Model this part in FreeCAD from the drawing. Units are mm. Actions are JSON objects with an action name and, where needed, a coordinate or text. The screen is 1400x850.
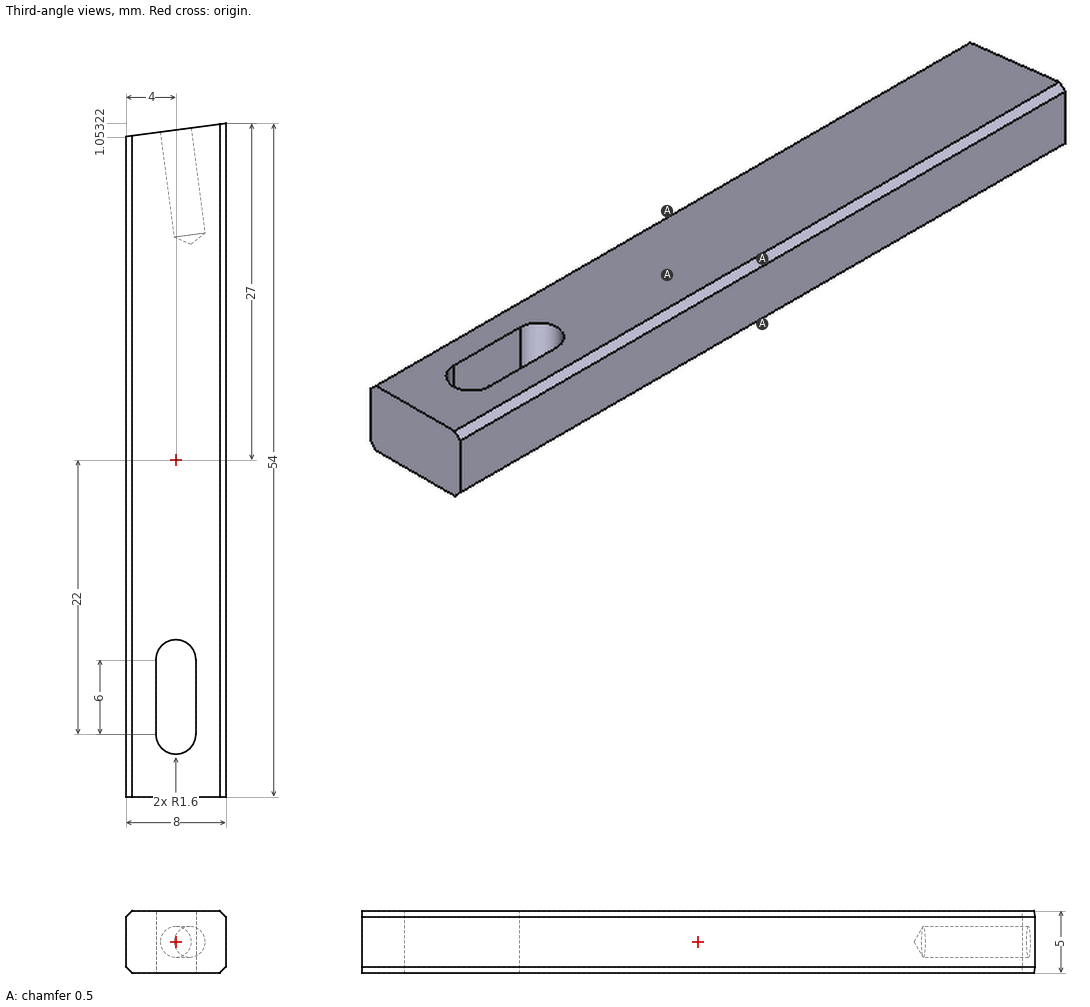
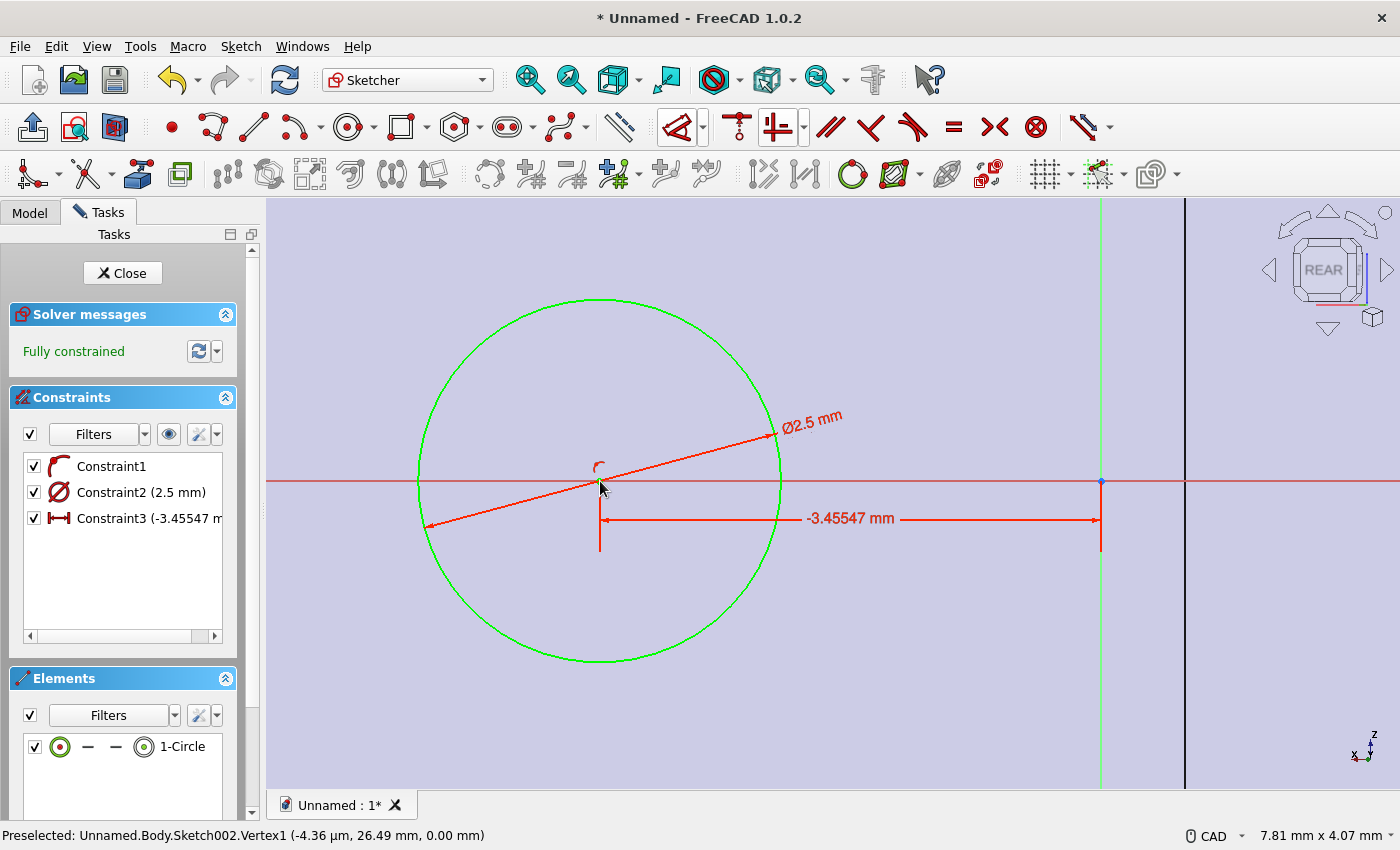
{"action": "left_click", "coordinate": [123, 273]}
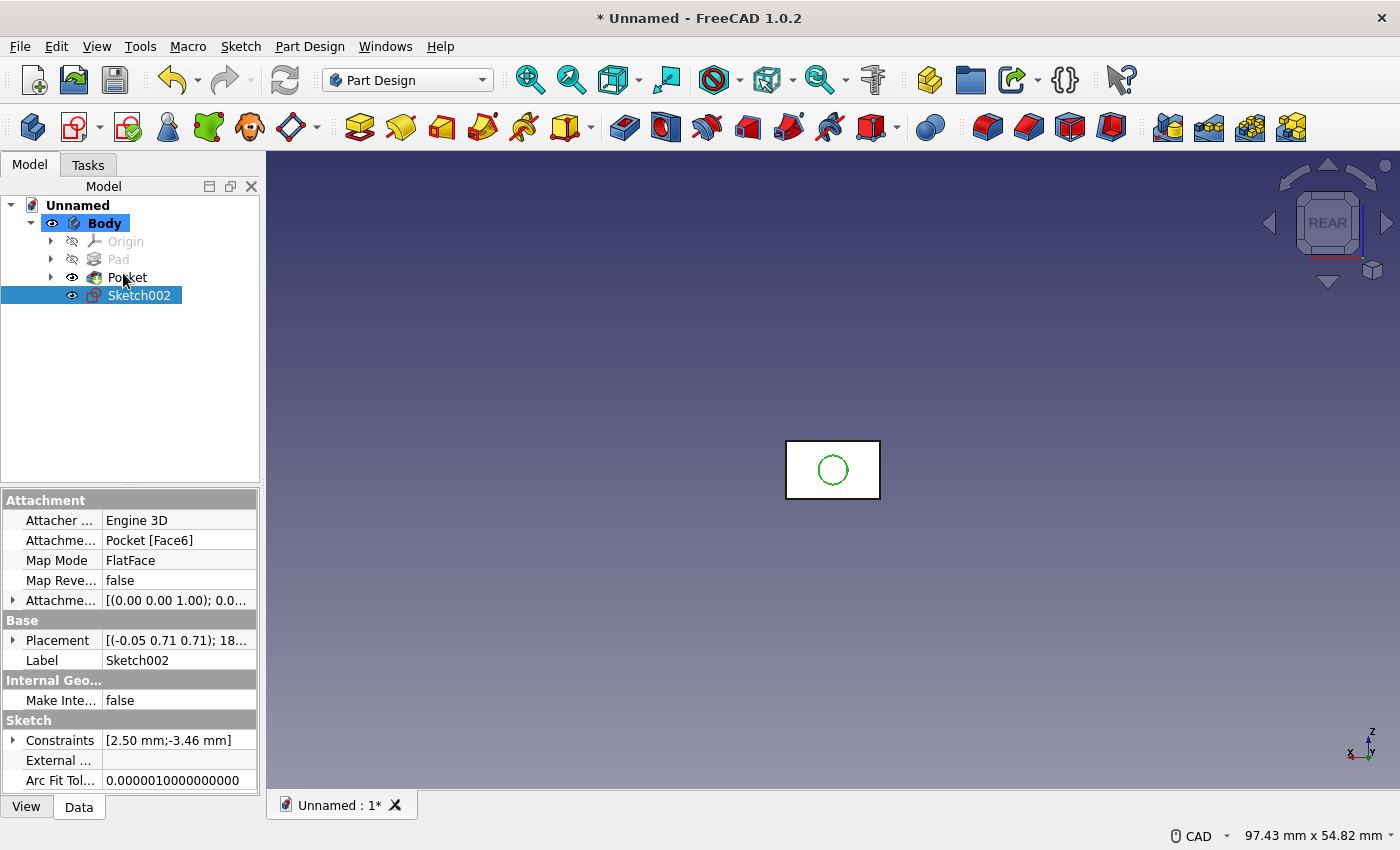
{"action": "left_click", "coordinate": [666, 128]}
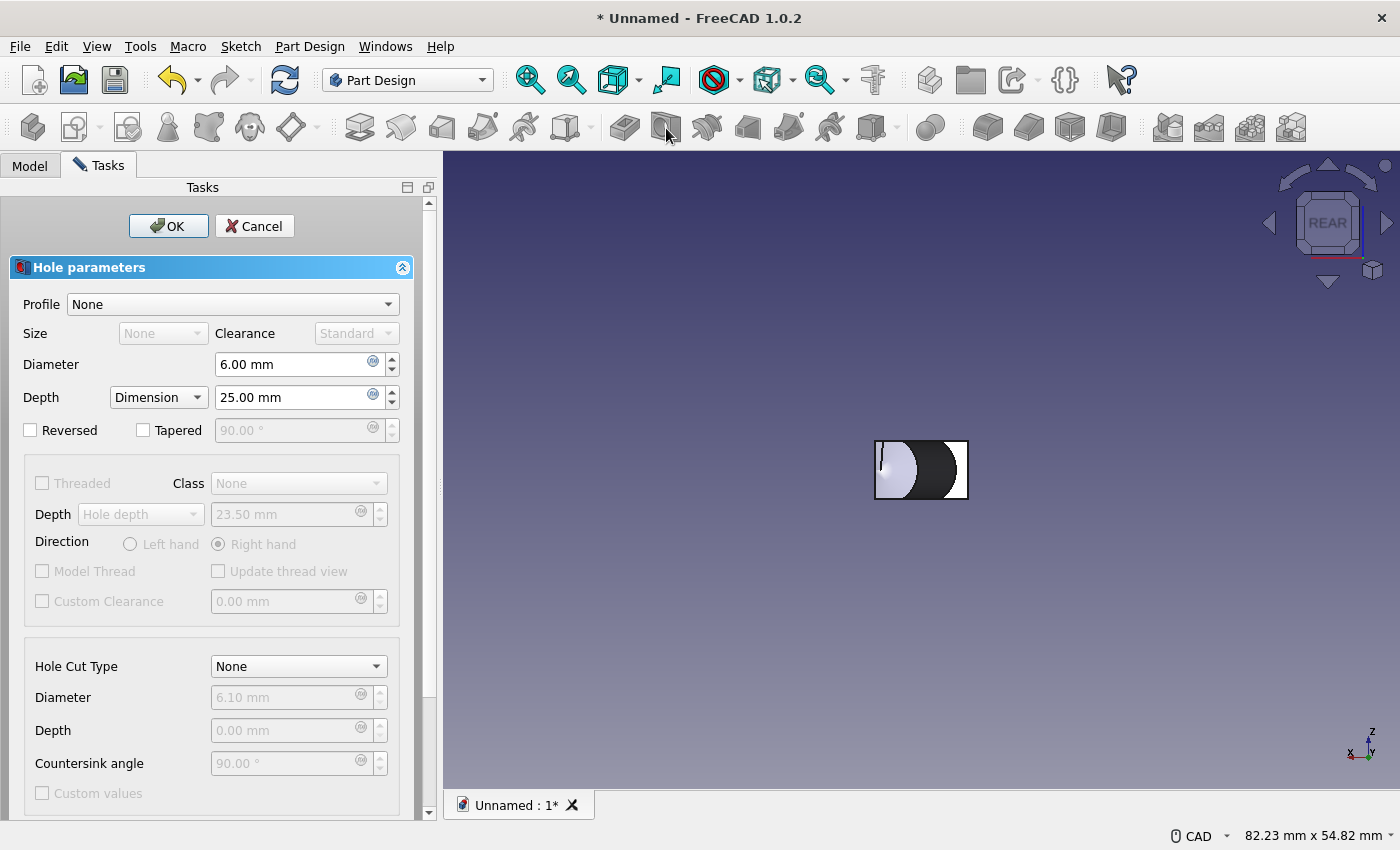
{"action": "triple_click", "coordinate": [300, 364]}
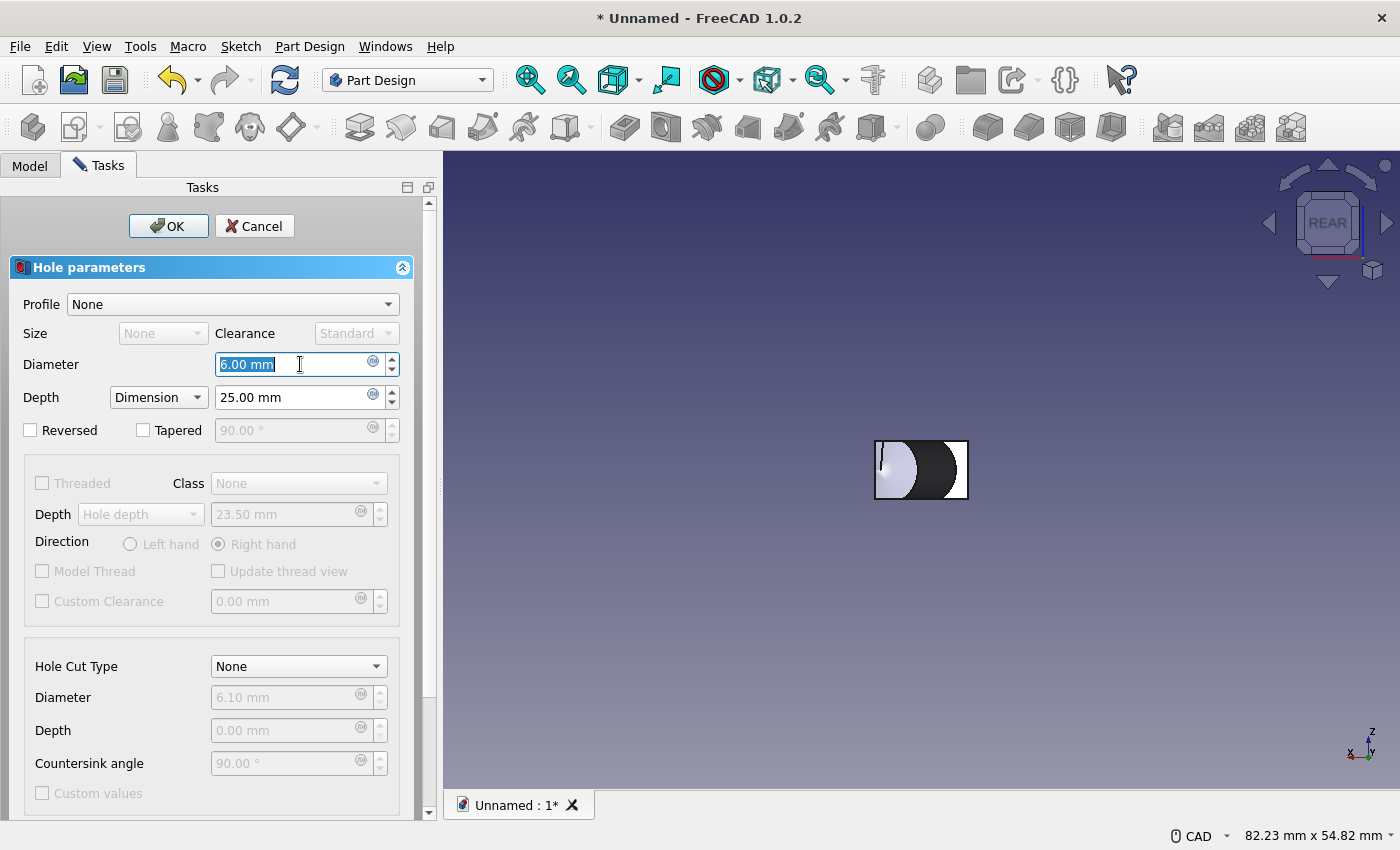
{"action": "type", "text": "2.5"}
{"action": "key", "text": "Tab"}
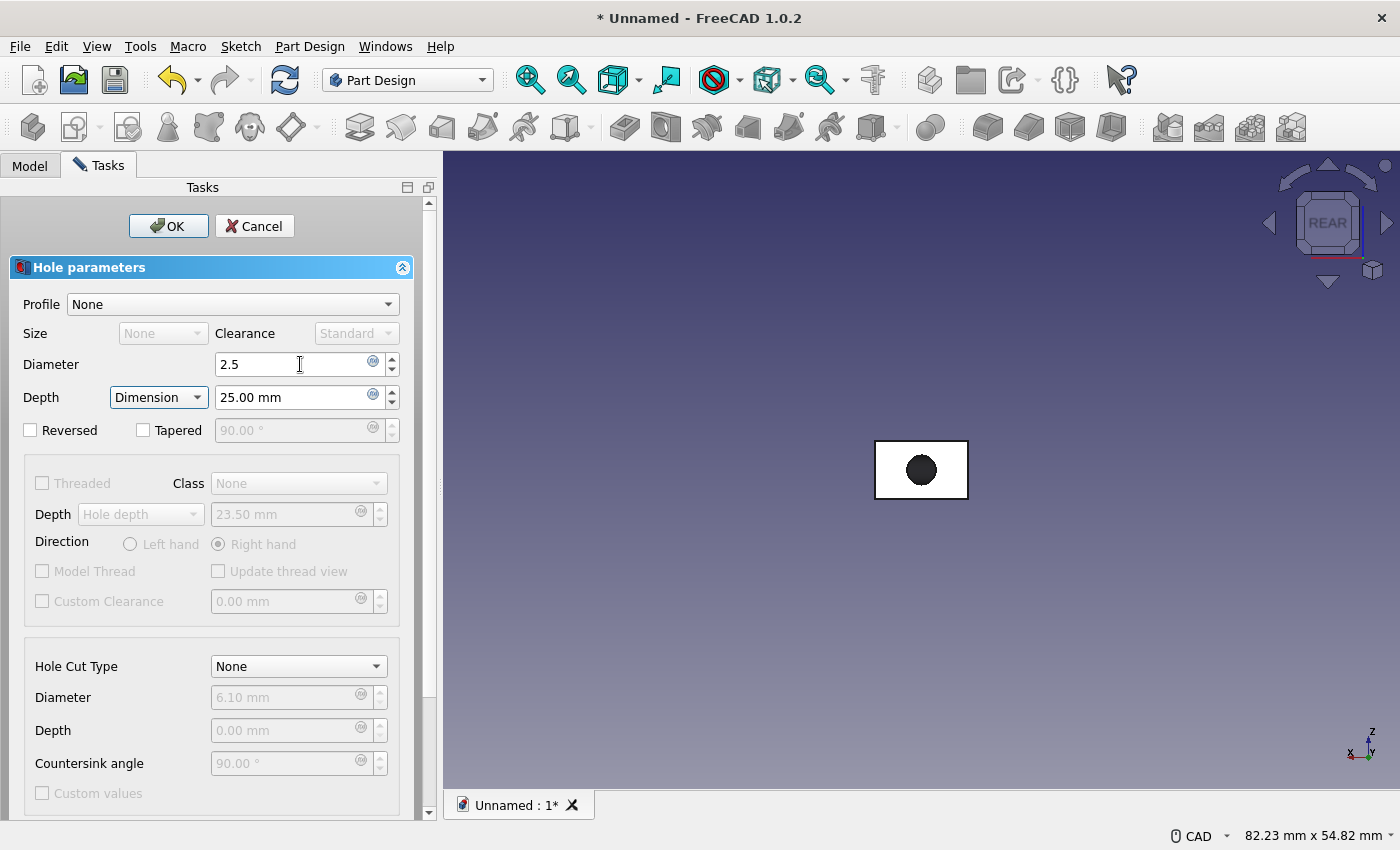
{"action": "triple_click", "coordinate": [300, 398]}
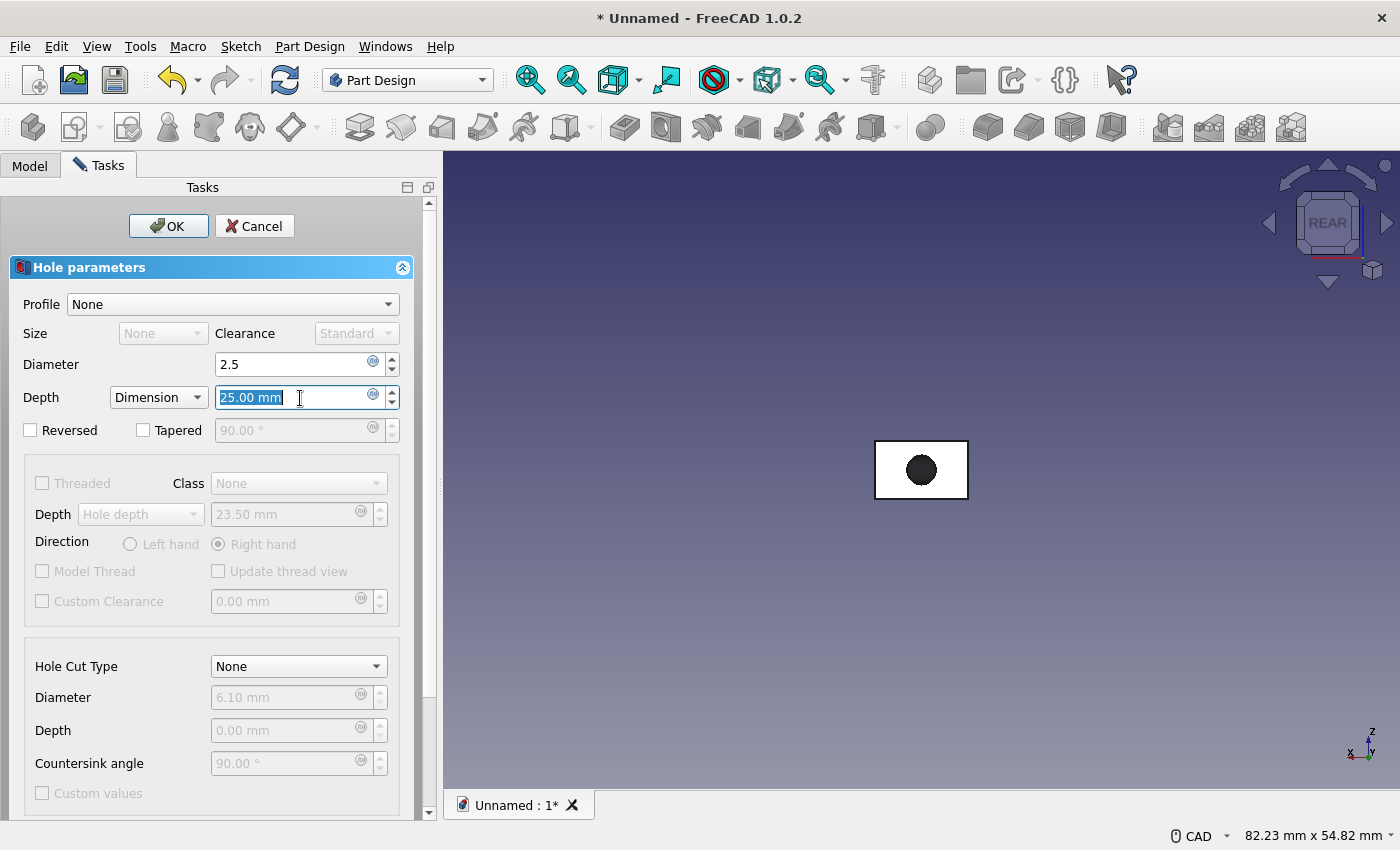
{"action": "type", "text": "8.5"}
{"action": "key", "text": "Tab"}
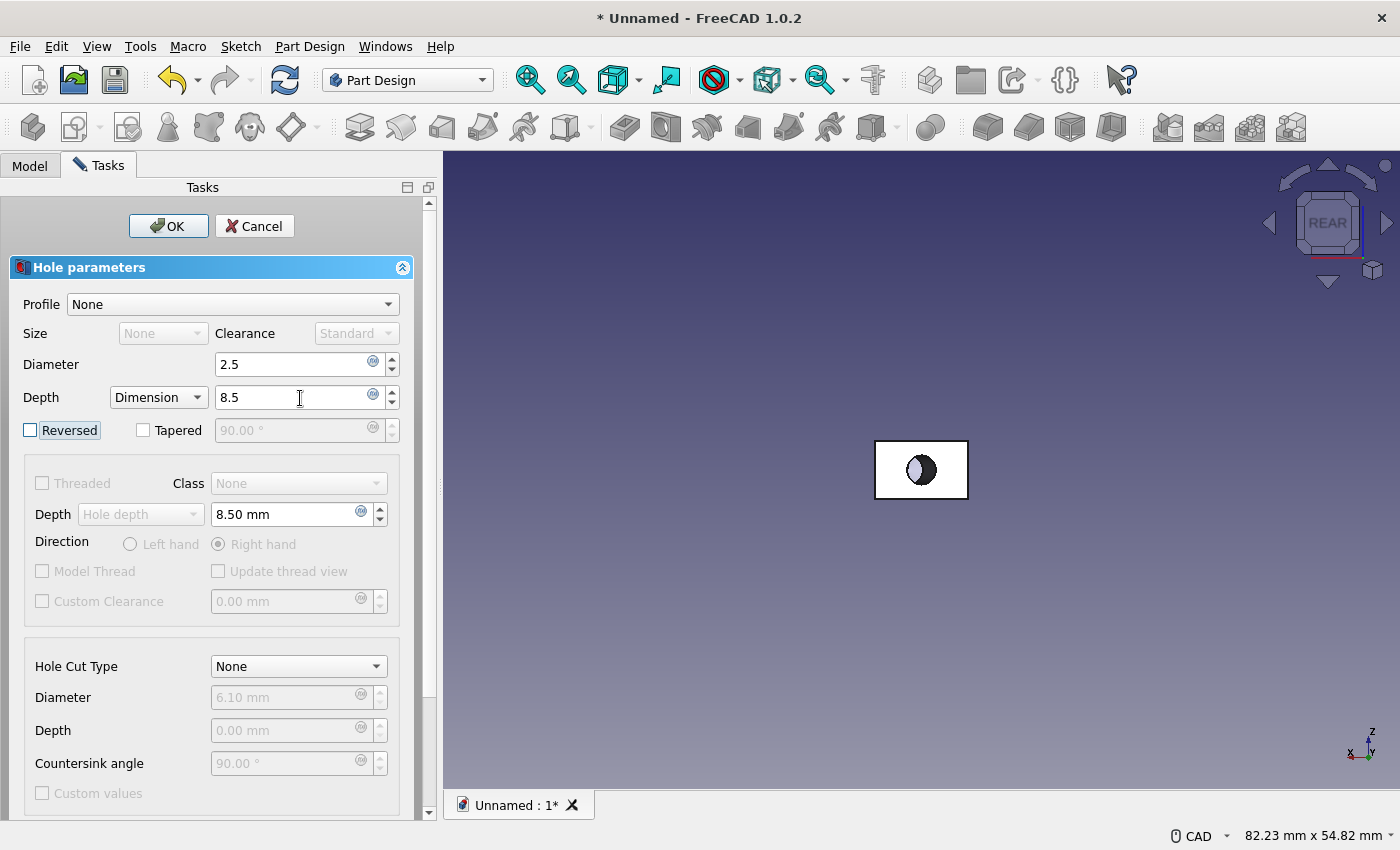
{"action": "left_click", "coordinate": [169, 226]}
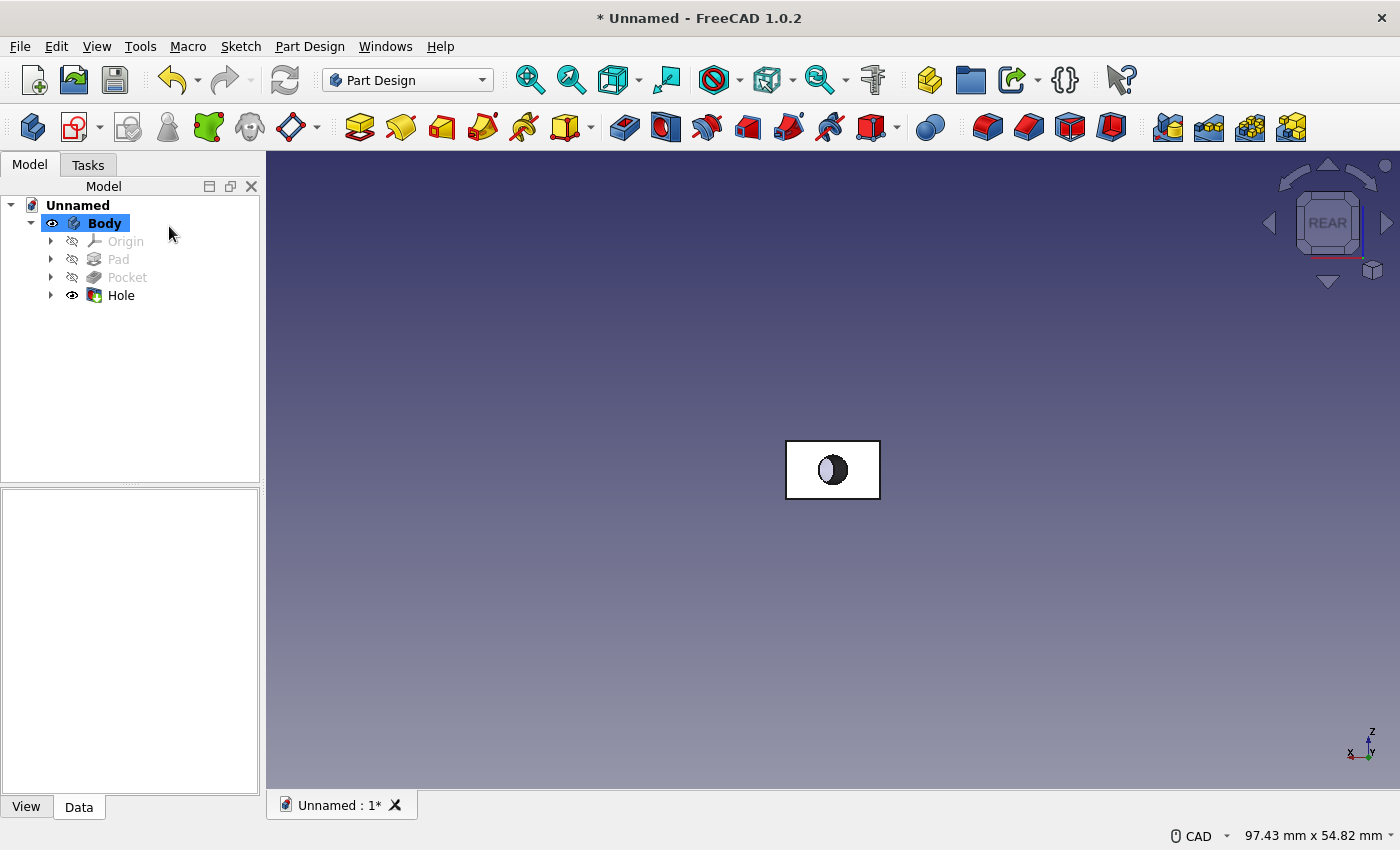
{"action": "key", "text": "v f"}